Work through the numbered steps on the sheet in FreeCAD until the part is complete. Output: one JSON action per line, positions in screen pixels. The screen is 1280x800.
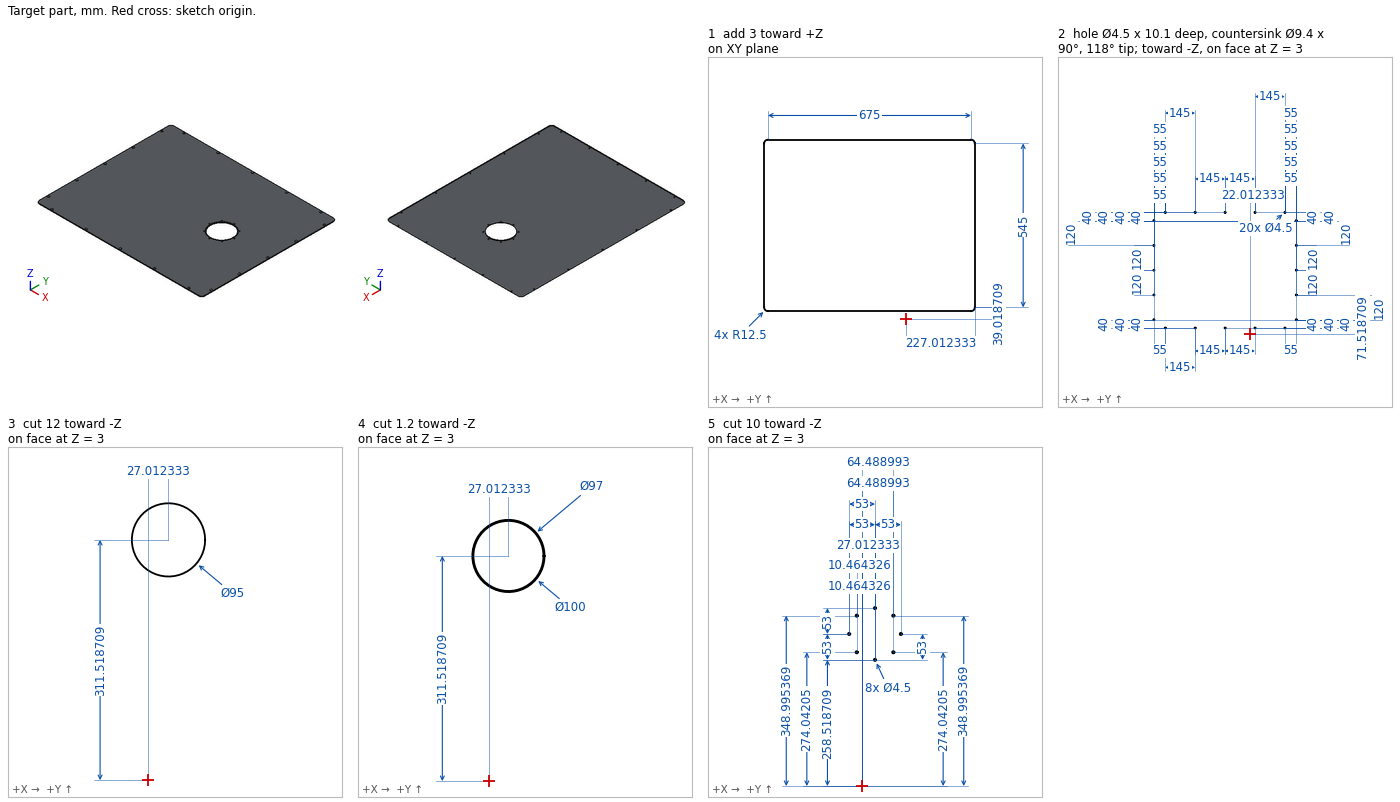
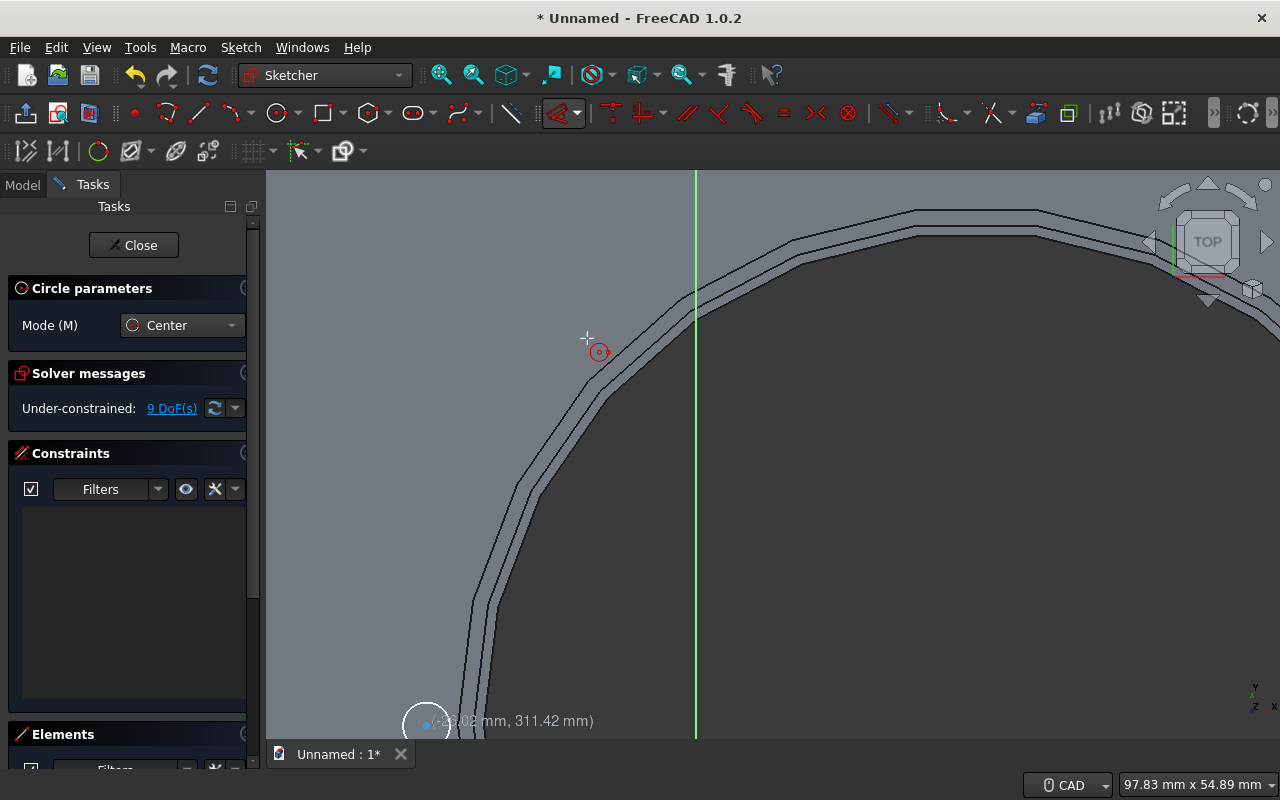
{"action": "left_click", "coordinate": [588, 336]}
{"action": "left_click", "coordinate": [604, 320]}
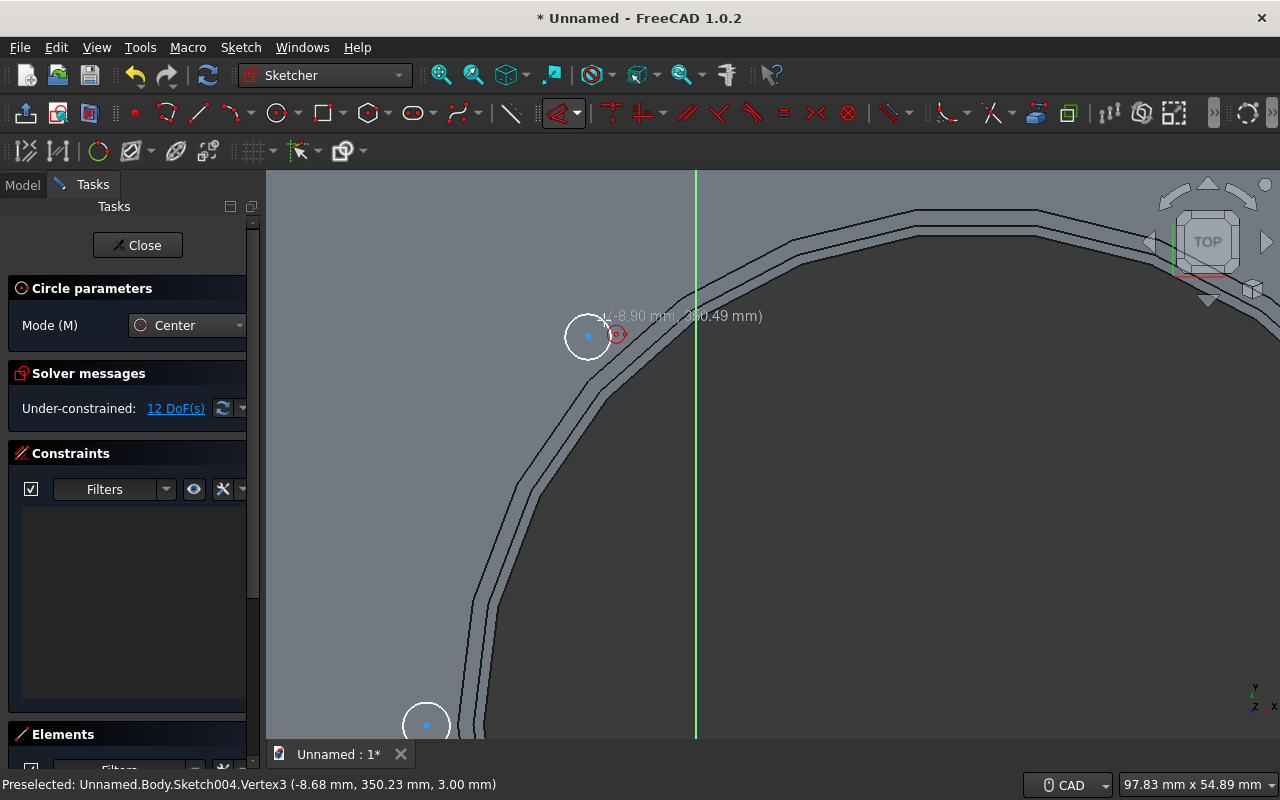
{"action": "scroll", "coordinate": [587, 338], "scroll_direction": "down", "scroll_amount": 6}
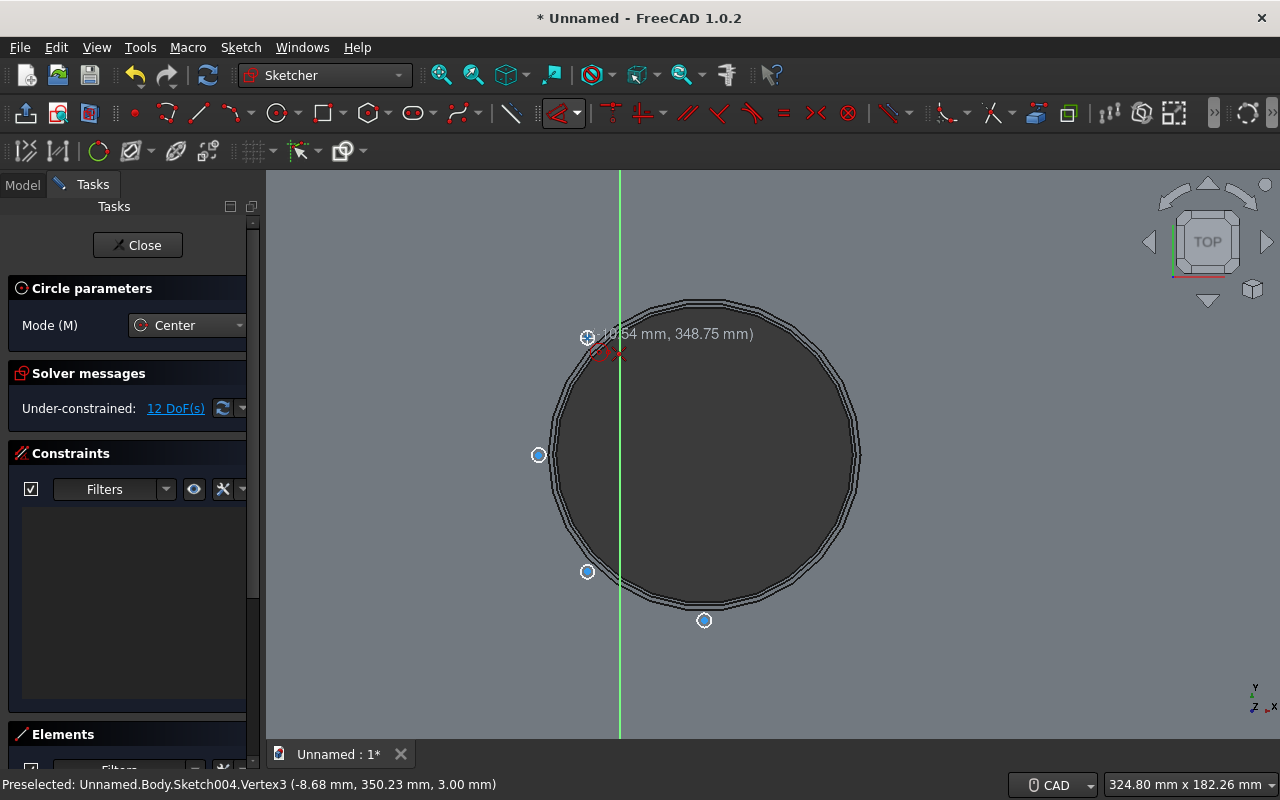
{"action": "scroll", "coordinate": [704, 289], "scroll_direction": "up", "scroll_amount": 6}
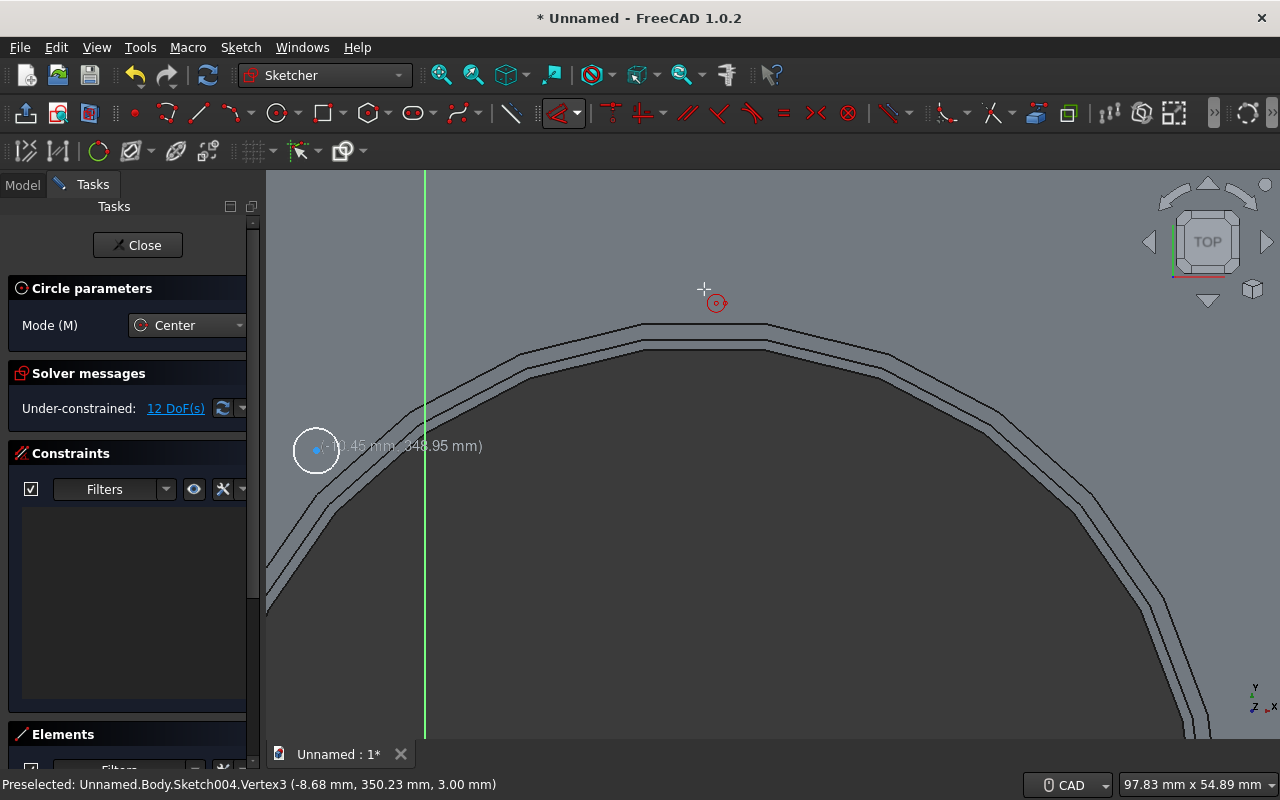
{"action": "left_click", "coordinate": [705, 289]}
{"action": "left_click", "coordinate": [721, 273]}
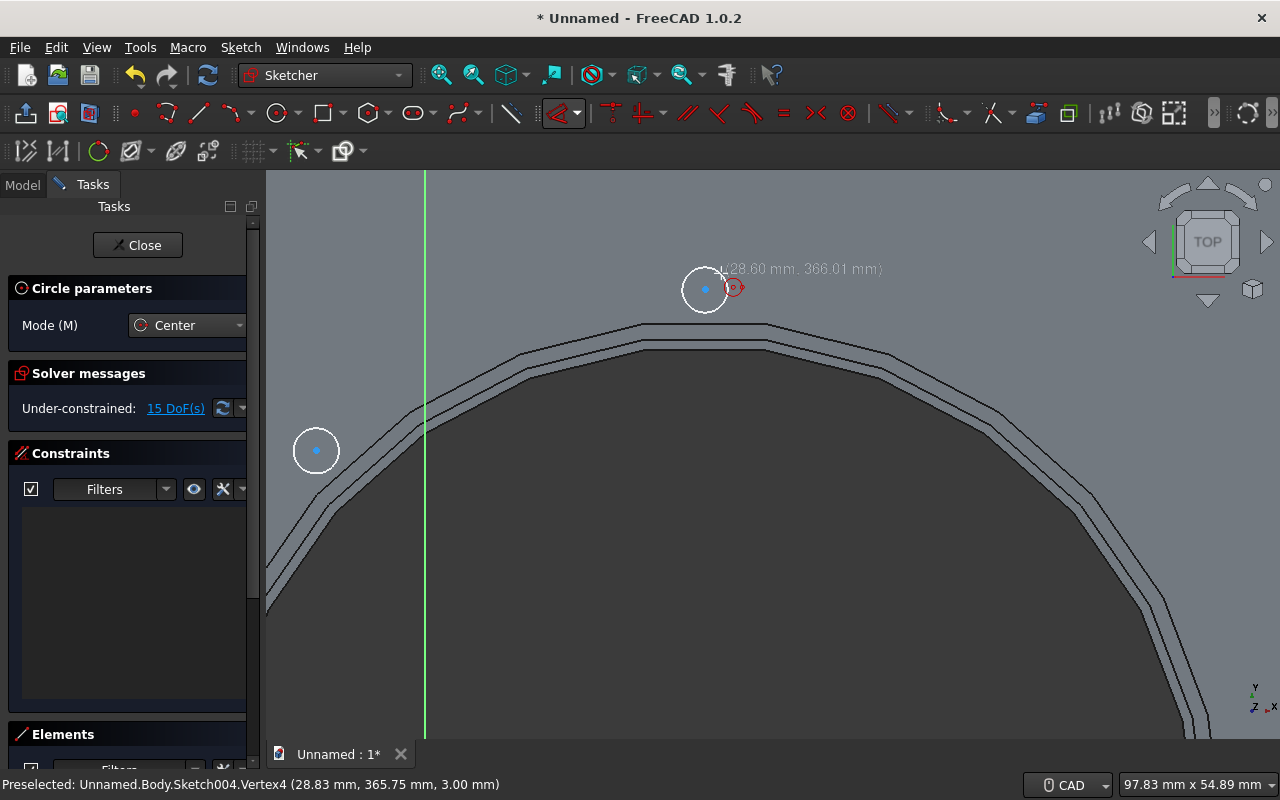
{"action": "left_click", "coordinate": [1093, 450]}
{"action": "left_click", "coordinate": [1109, 434]}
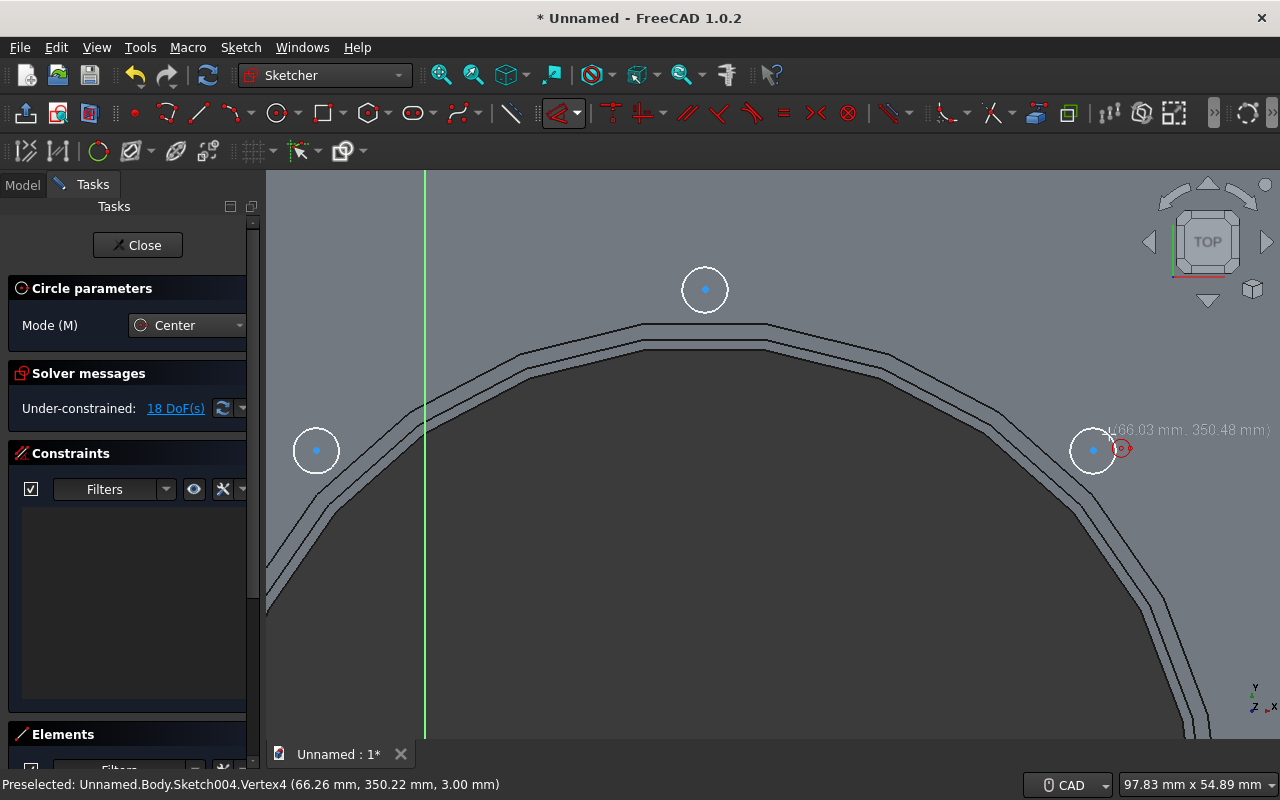
{"action": "scroll", "coordinate": [704, 289], "scroll_direction": "down", "scroll_amount": 6}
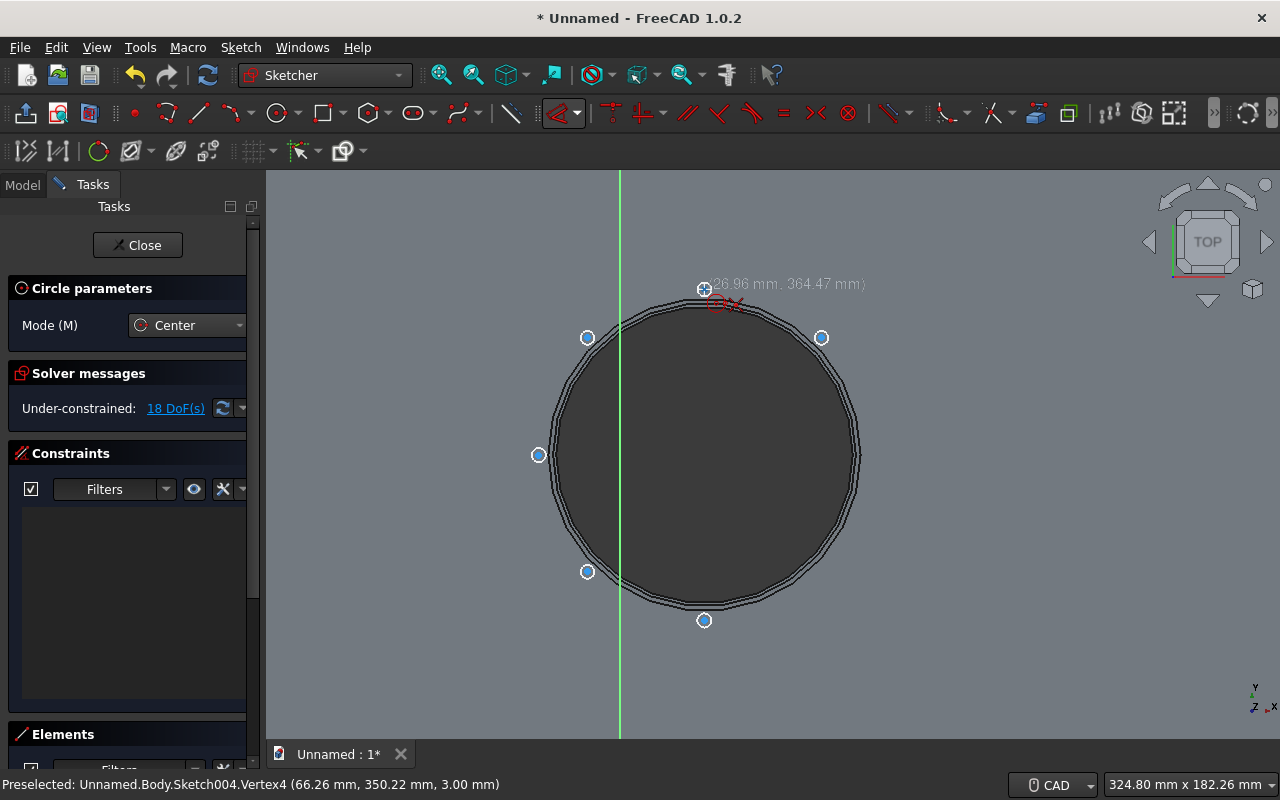
{"action": "scroll", "coordinate": [870, 455], "scroll_direction": "up", "scroll_amount": 6}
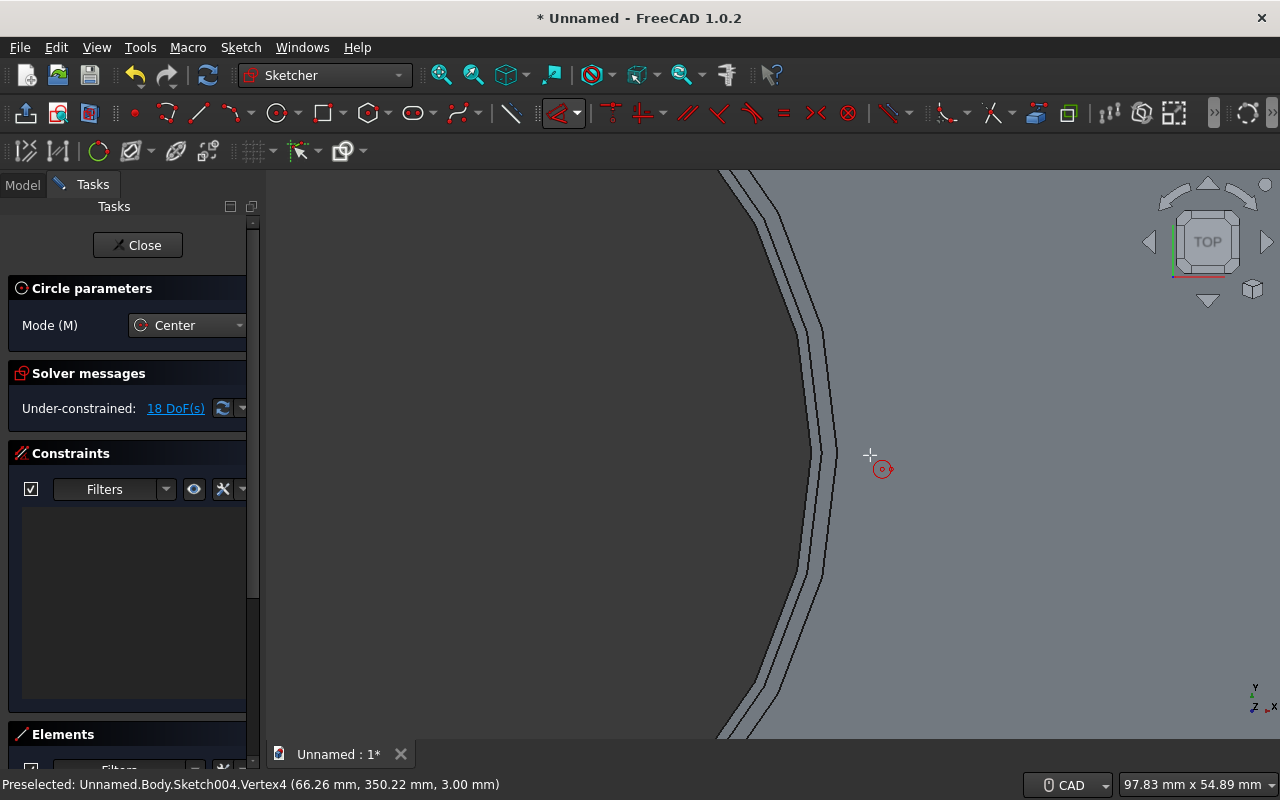
{"action": "left_click", "coordinate": [868, 453]}
{"action": "left_click", "coordinate": [885, 437]}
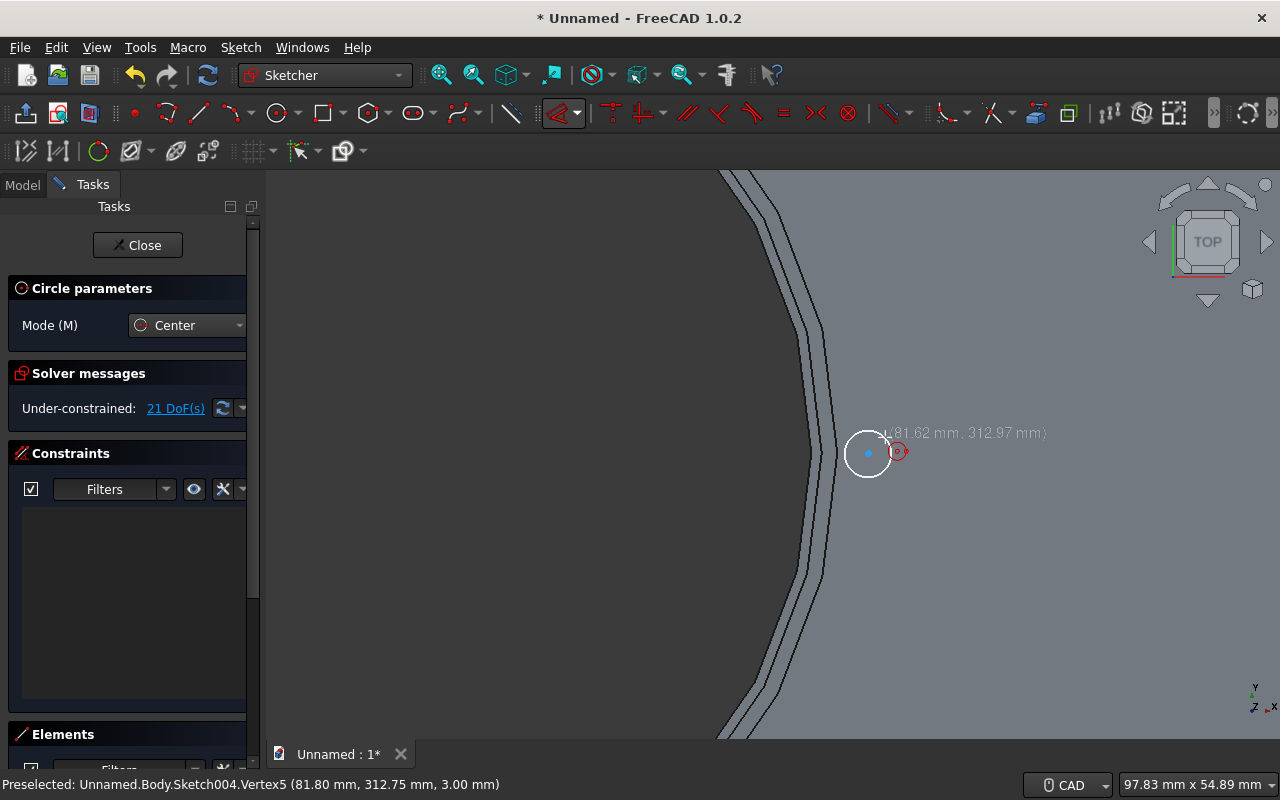
{"action": "scroll", "coordinate": [871, 455], "scroll_direction": "down", "scroll_amount": 6}